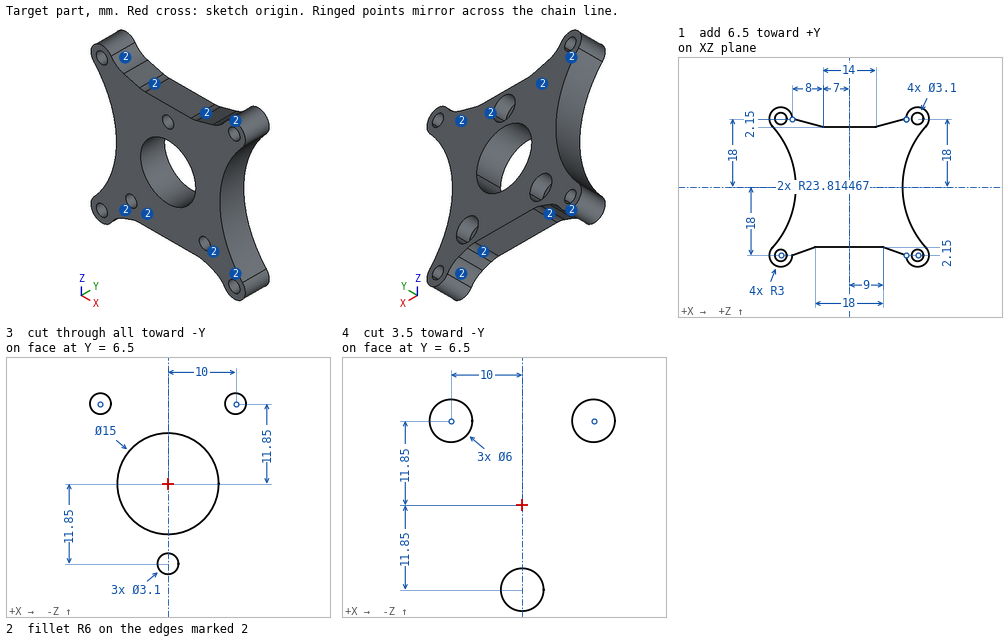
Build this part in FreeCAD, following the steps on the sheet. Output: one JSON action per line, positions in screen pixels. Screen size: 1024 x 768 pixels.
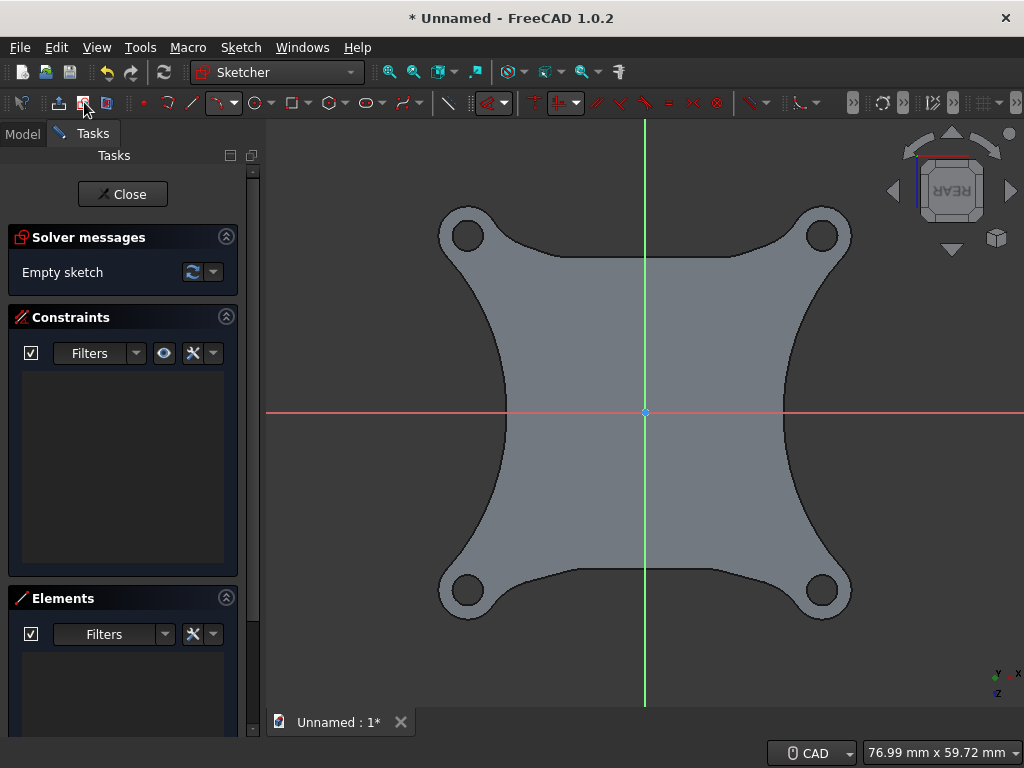
{"action": "scroll", "coordinate": [784, 413], "scroll_direction": "up", "scroll_amount": 2}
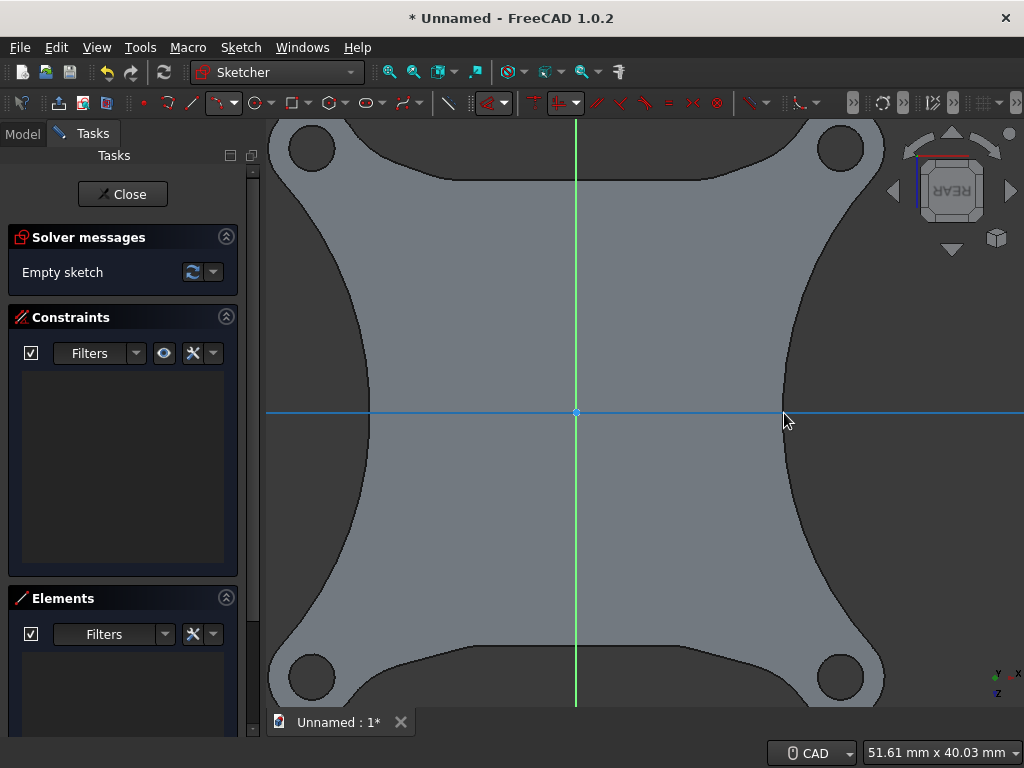
{"action": "left_click", "coordinate": [256, 104]}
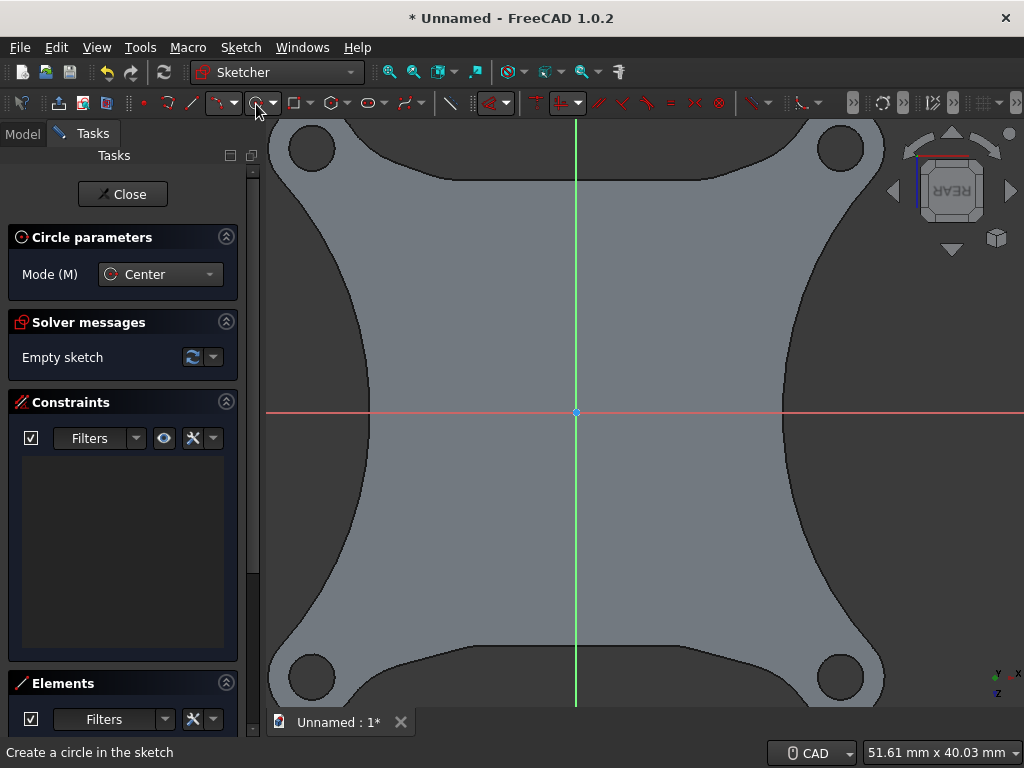
{"action": "left_click", "coordinate": [576, 413]}
{"action": "left_click", "coordinate": [654, 335]}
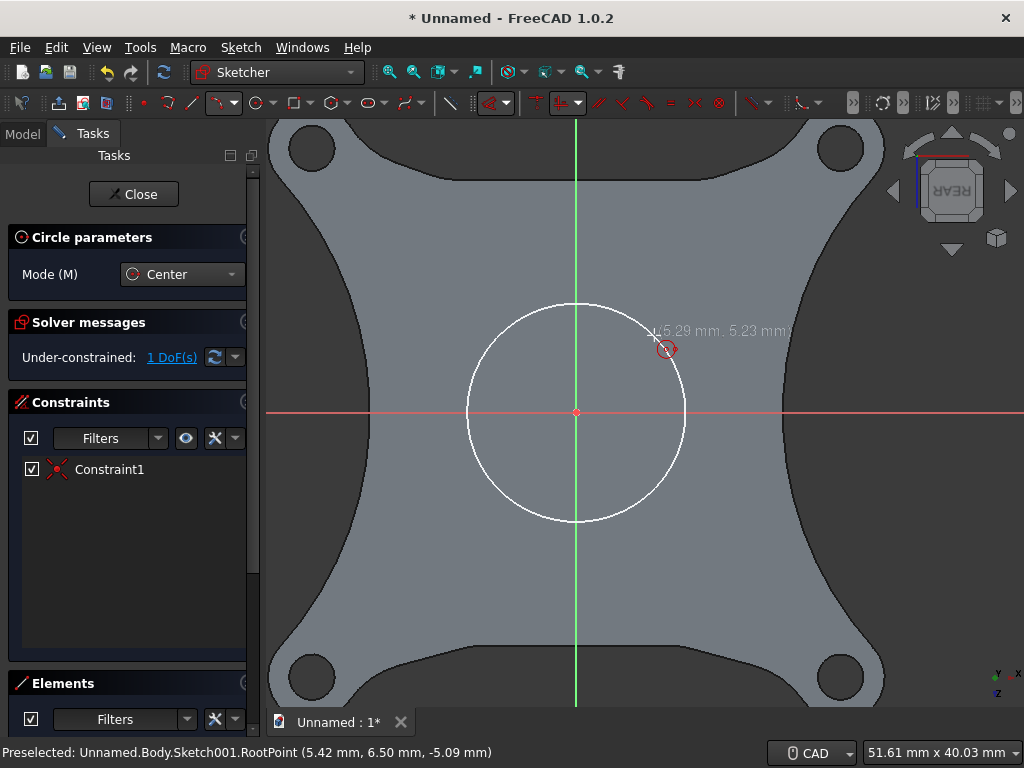
{"action": "left_click", "coordinate": [723, 239]}
{"action": "left_click", "coordinate": [739, 223]}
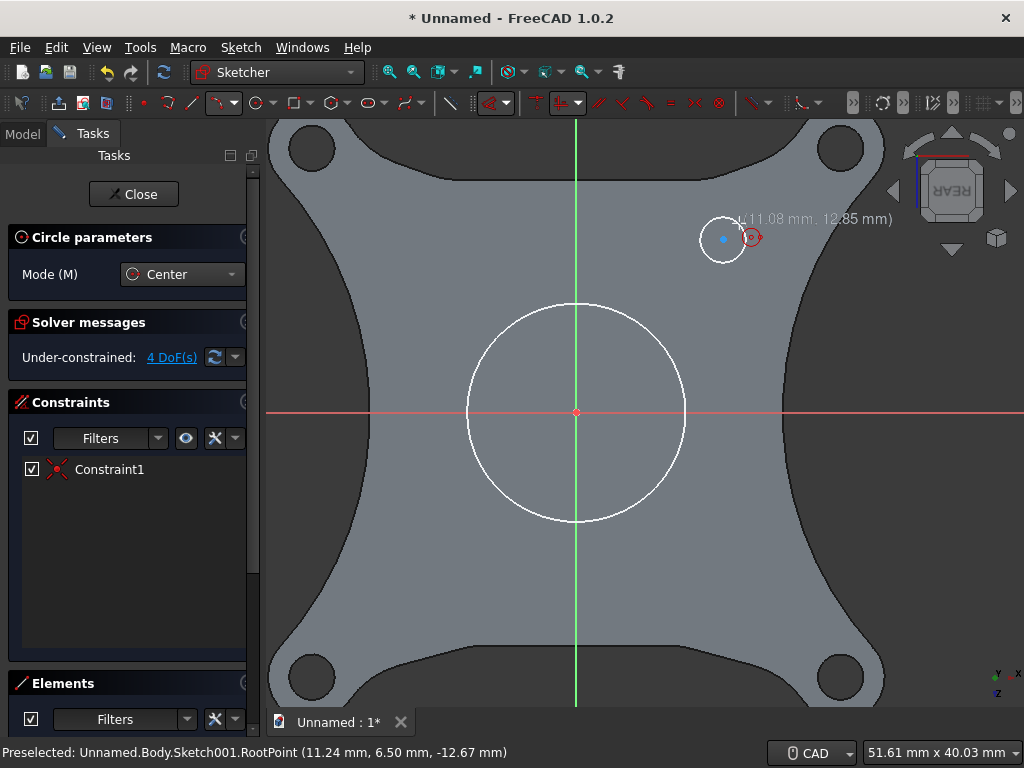
{"action": "left_click", "coordinate": [576, 587]}
{"action": "left_click", "coordinate": [592, 571]}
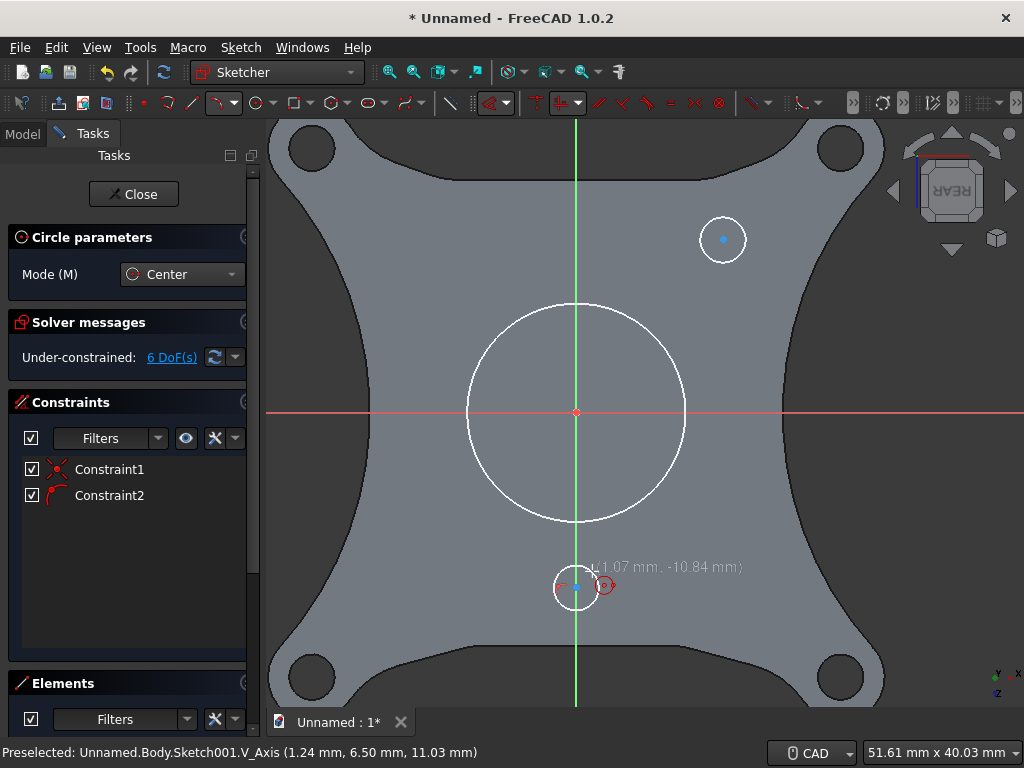
{"action": "left_click", "coordinate": [429, 239]}
{"action": "left_click", "coordinate": [446, 223]}
{"action": "key", "text": "Escape"}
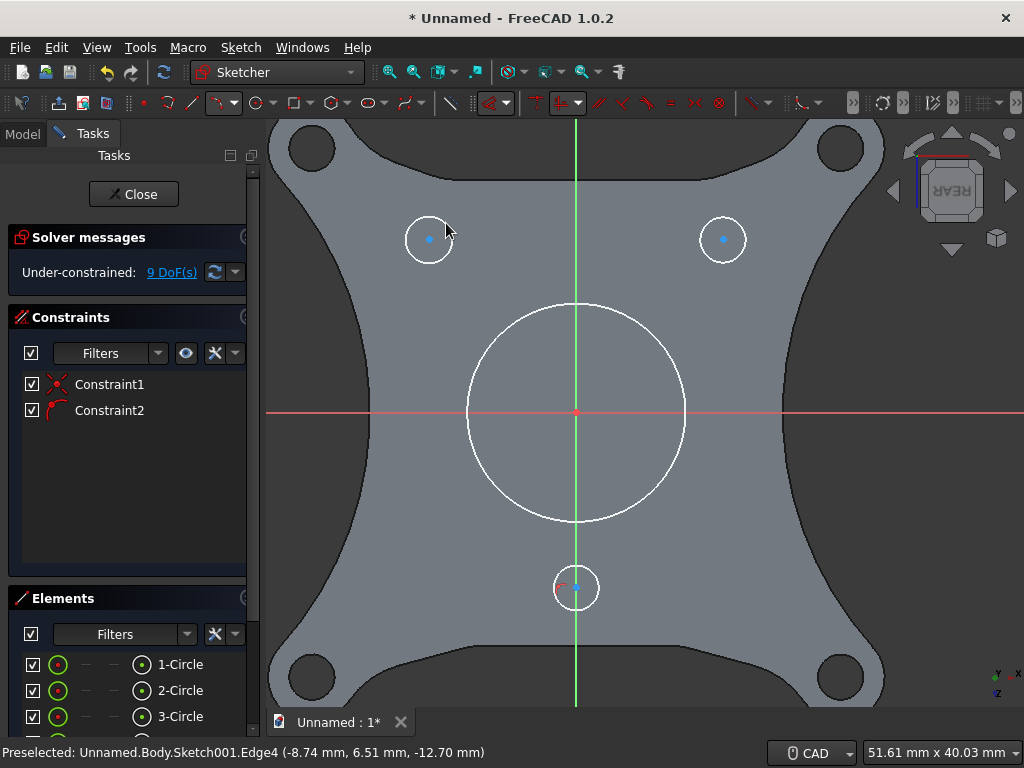
{"action": "left_click", "coordinate": [739, 224]}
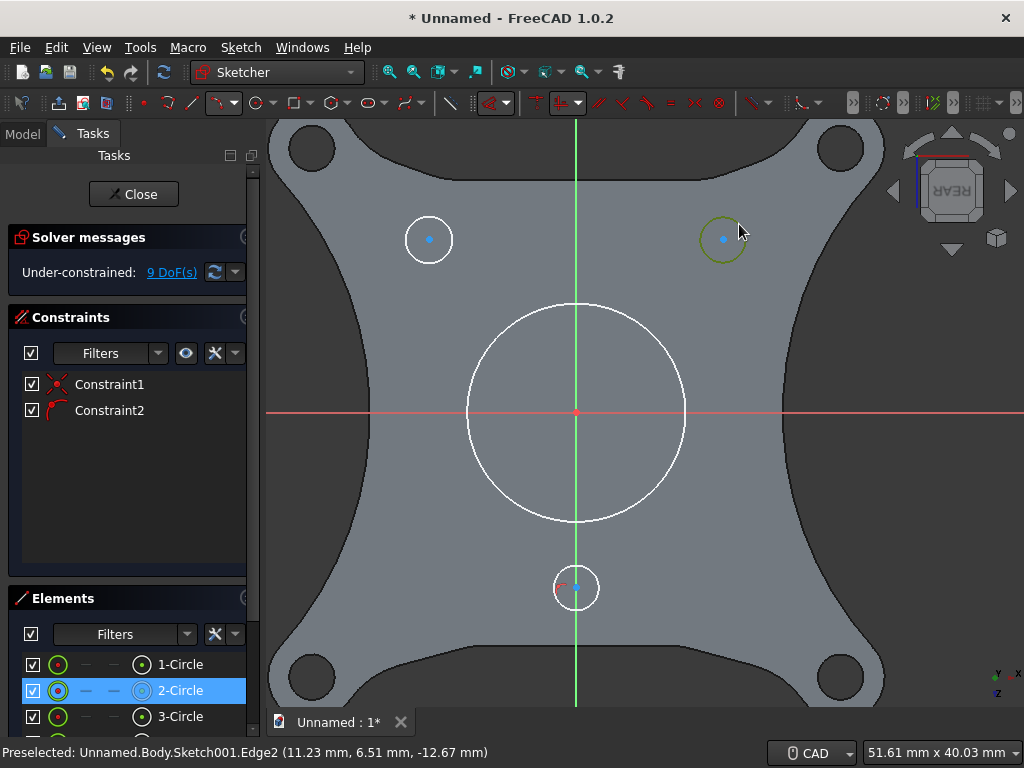
{"action": "left_click", "coordinate": [592, 572]}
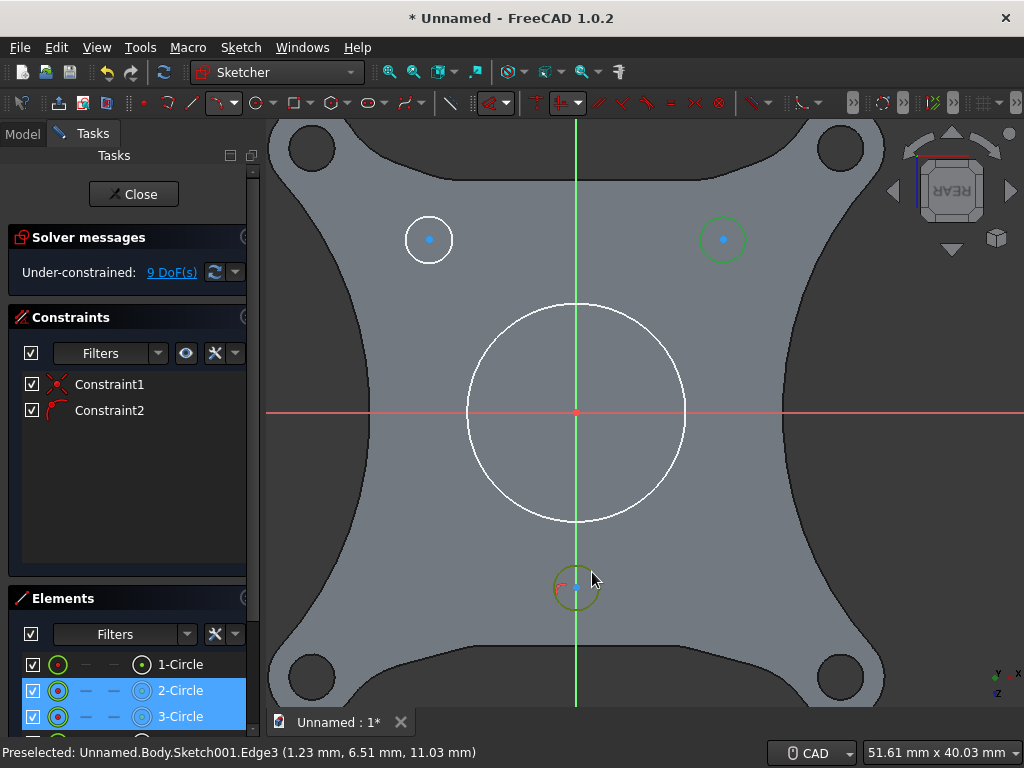
{"action": "left_click", "coordinate": [445, 223]}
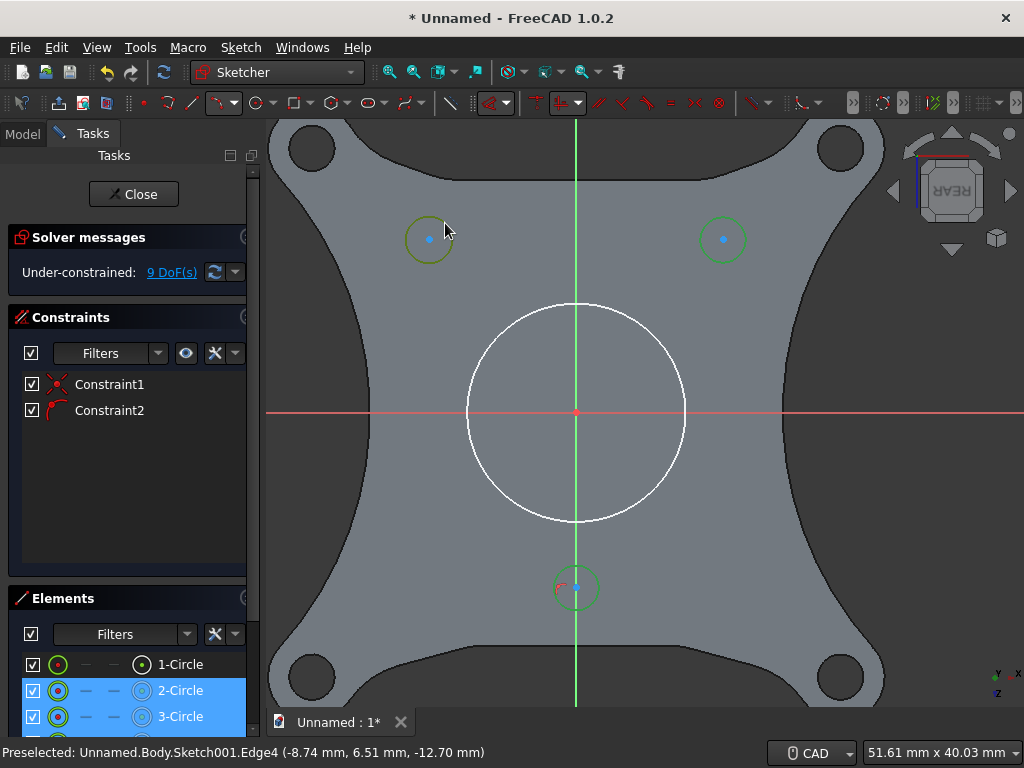
{"action": "left_click", "coordinate": [672, 104]}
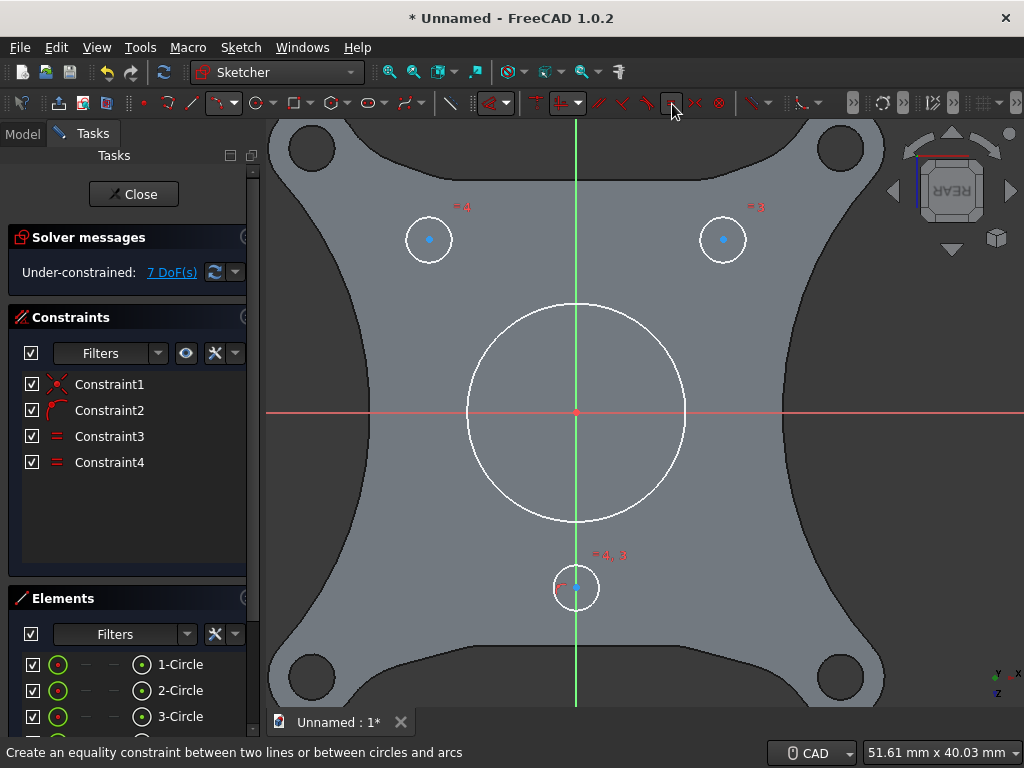
{"action": "left_click", "coordinate": [723, 240]}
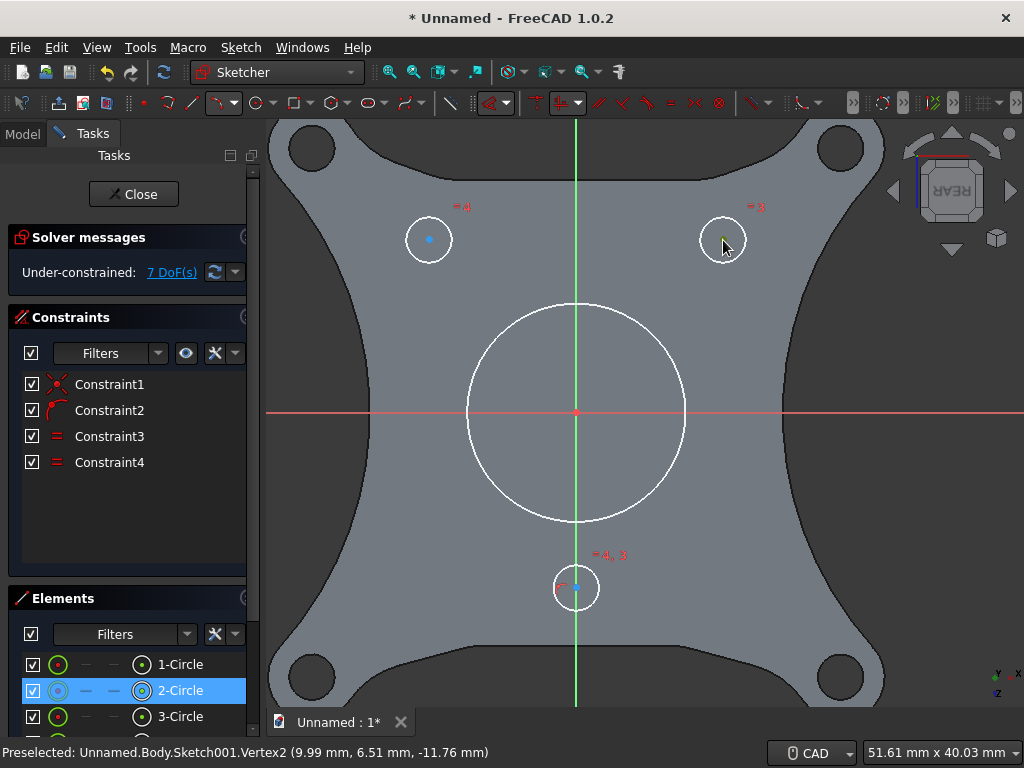
{"action": "left_click", "coordinate": [429, 240]}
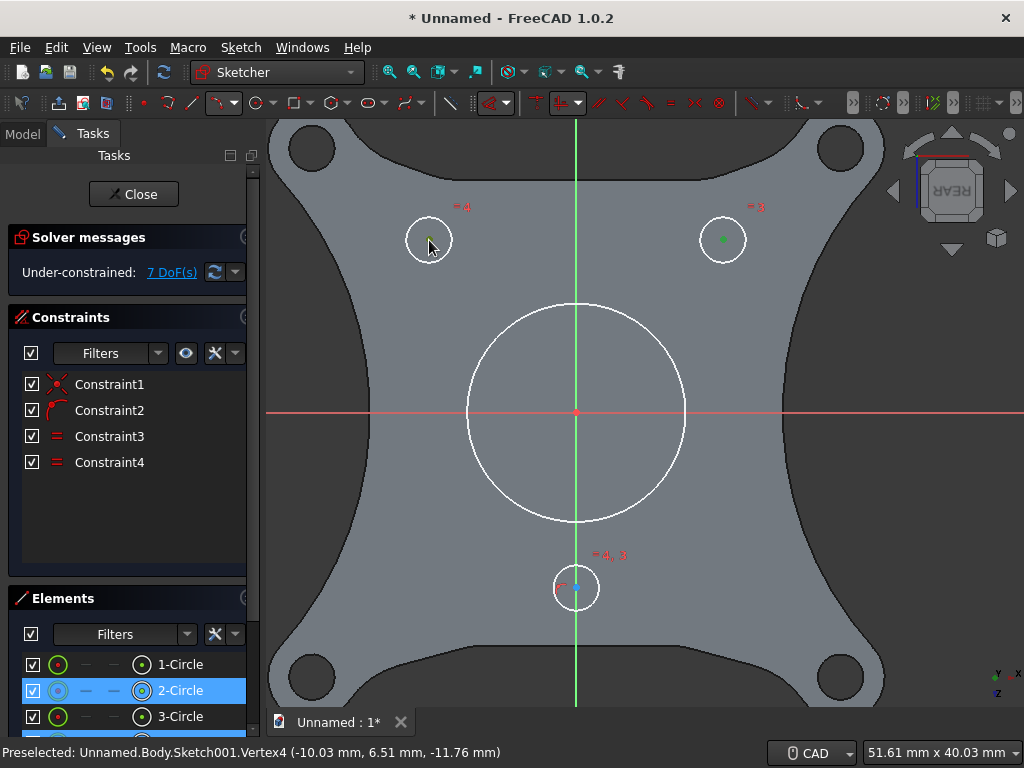
{"action": "left_click", "coordinate": [576, 641]}